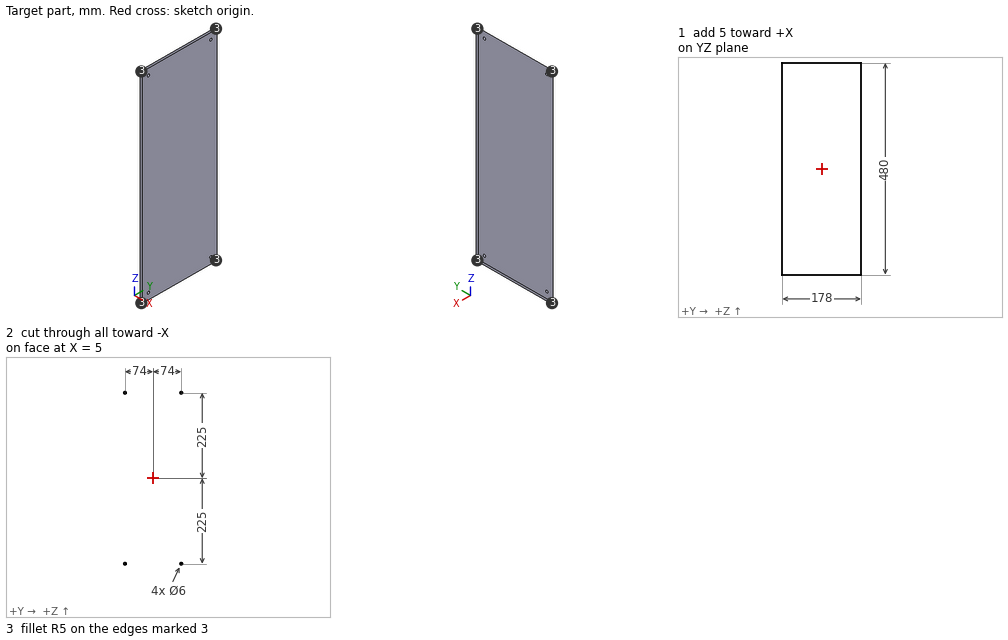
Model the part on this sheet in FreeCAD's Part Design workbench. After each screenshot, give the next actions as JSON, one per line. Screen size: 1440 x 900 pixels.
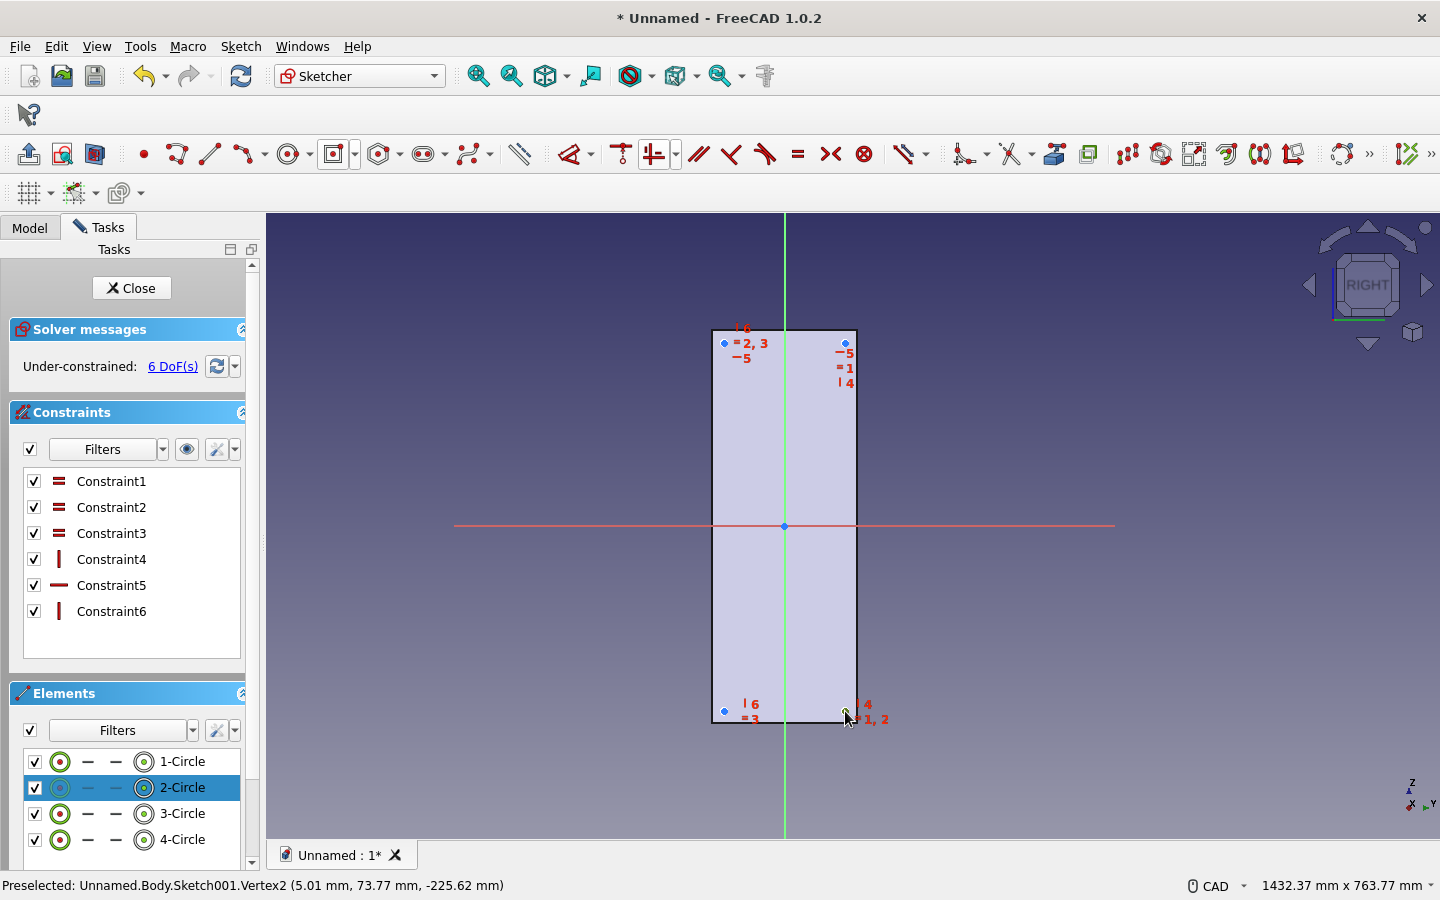
{"action": "left_click", "coordinate": [724, 711]}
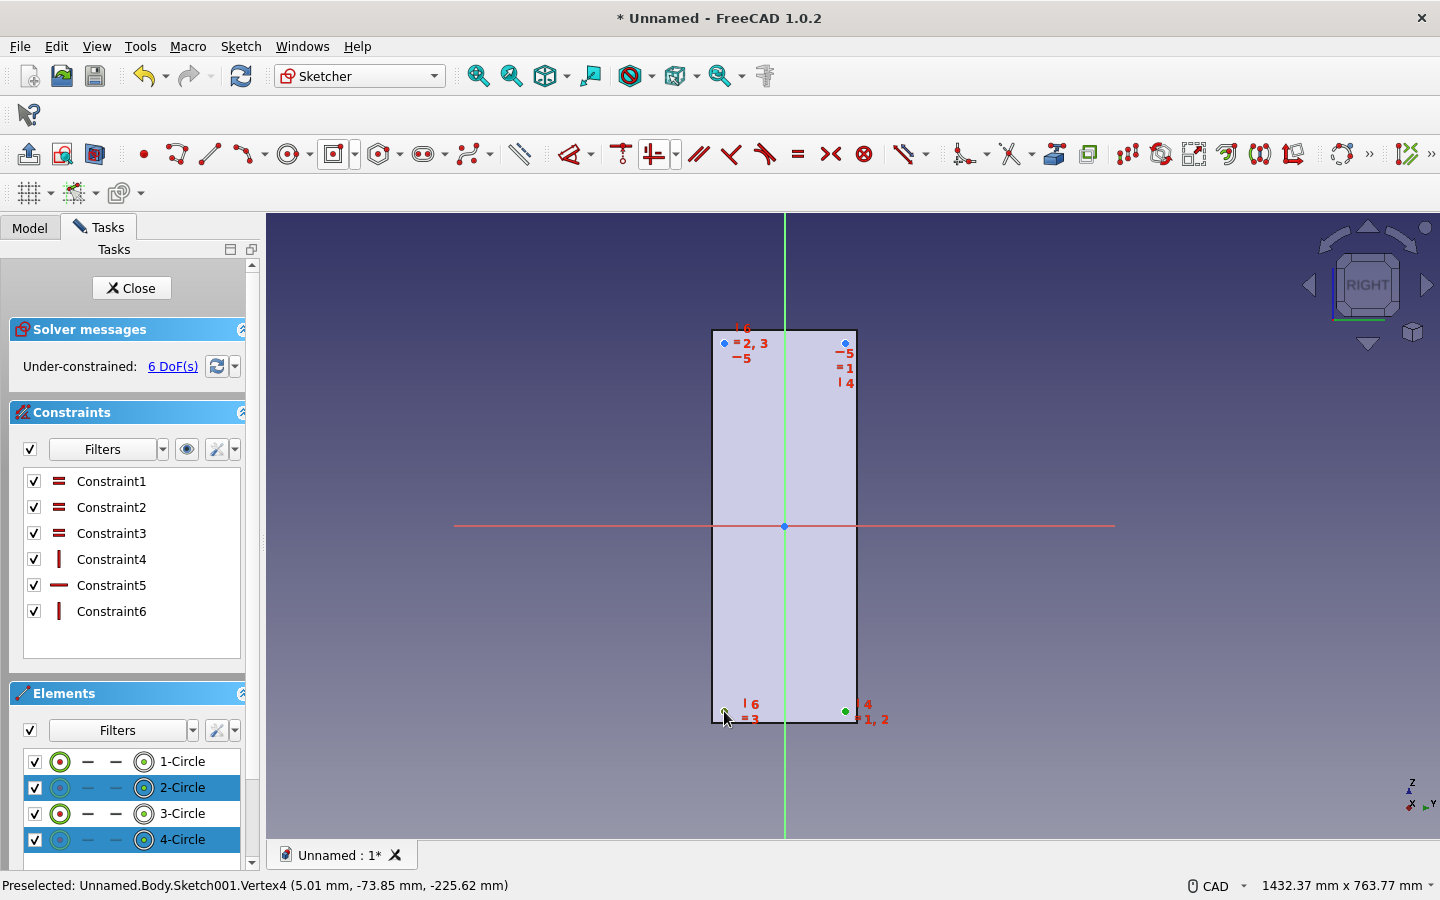
{"action": "key", "text": "h"}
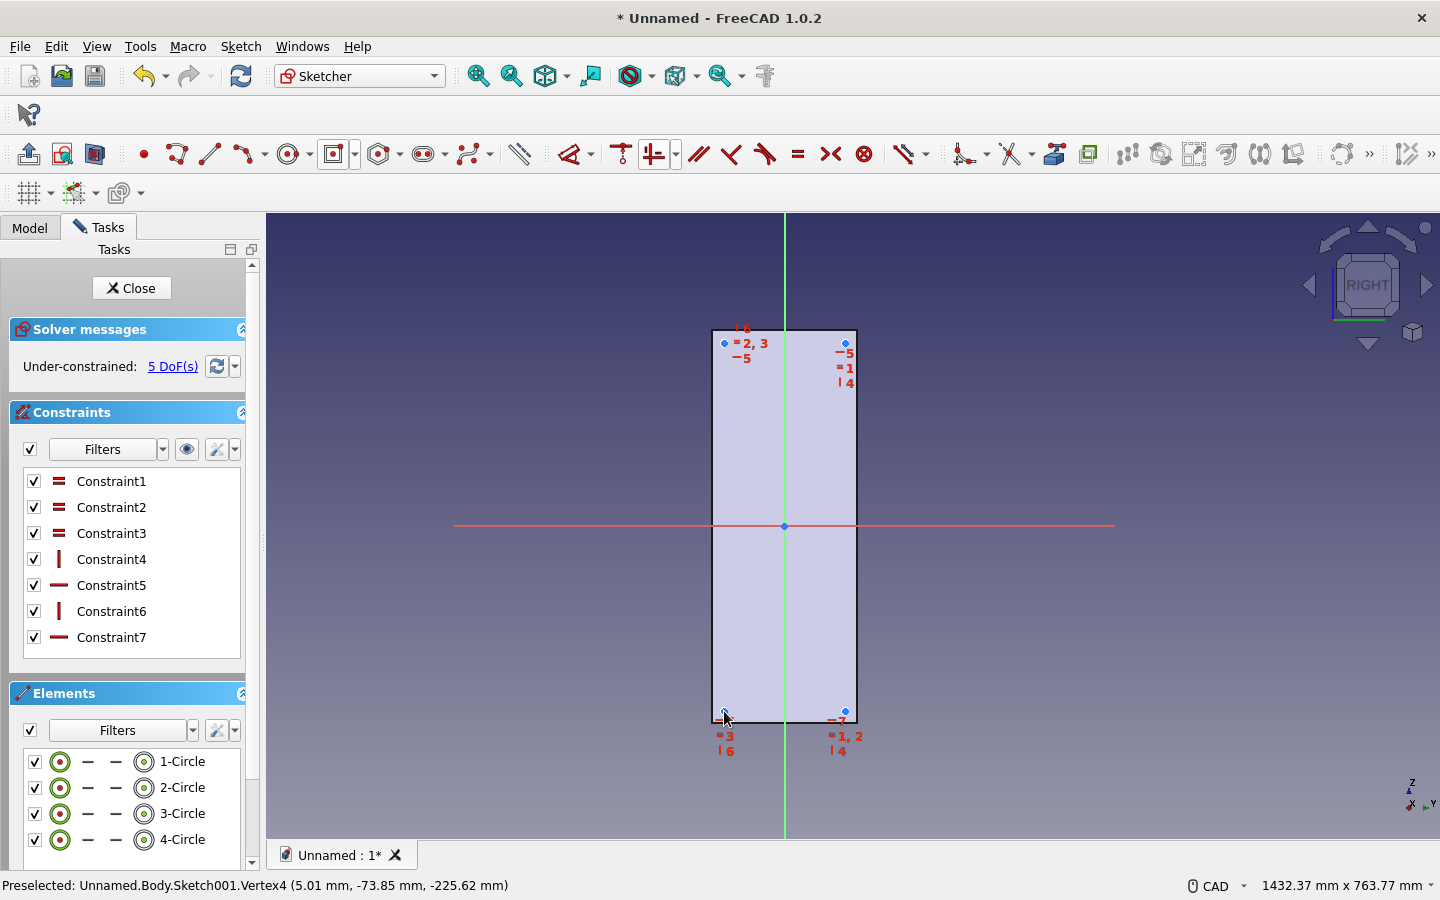
{"action": "scroll", "coordinate": [845, 340], "scroll_direction": "up", "scroll_amount": 11}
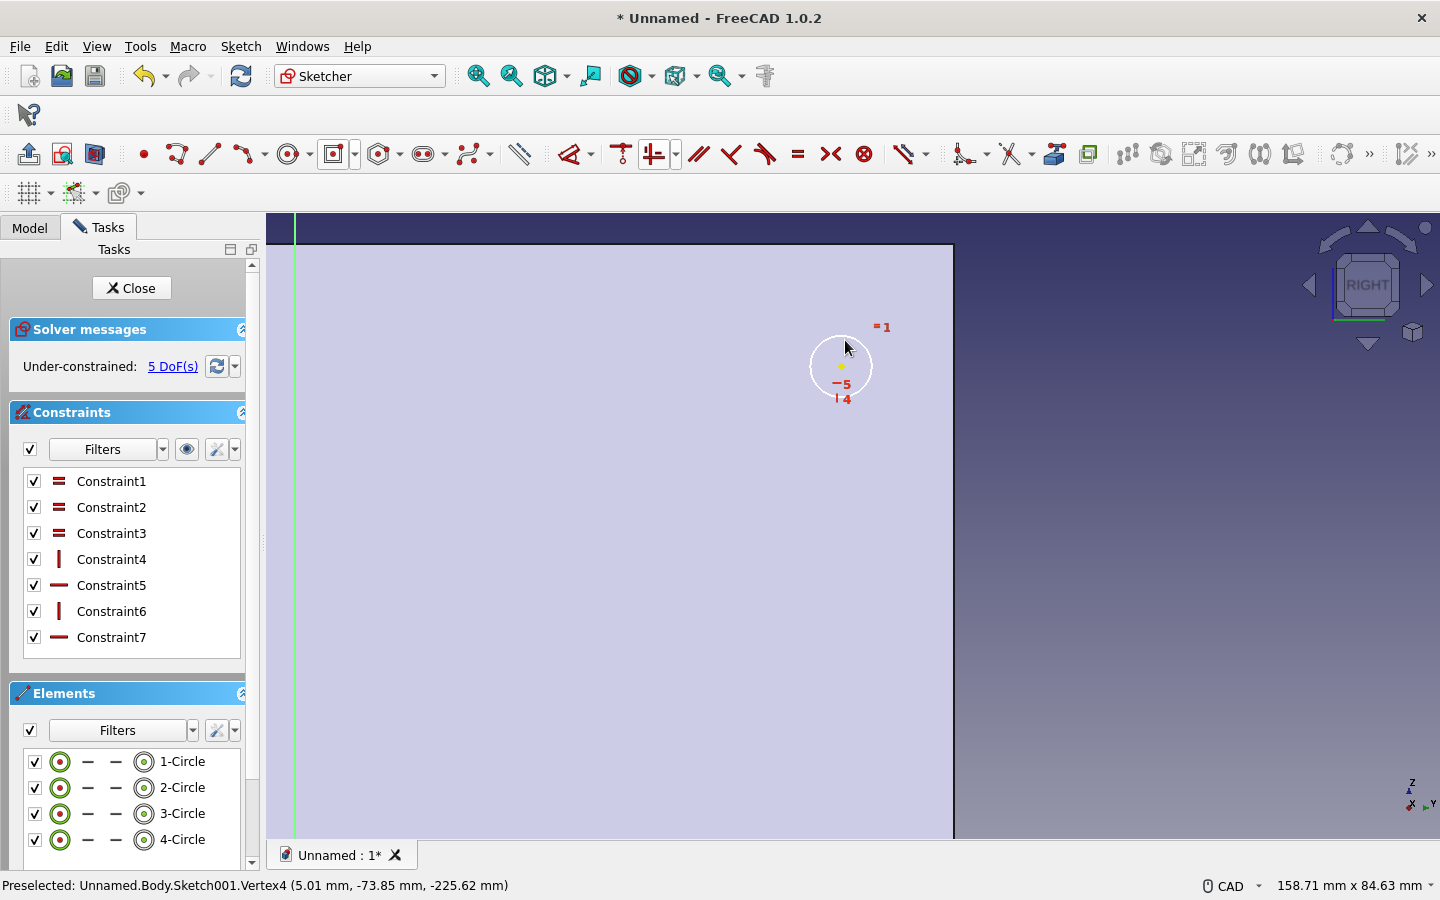
{"action": "left_click", "coordinate": [842, 336]}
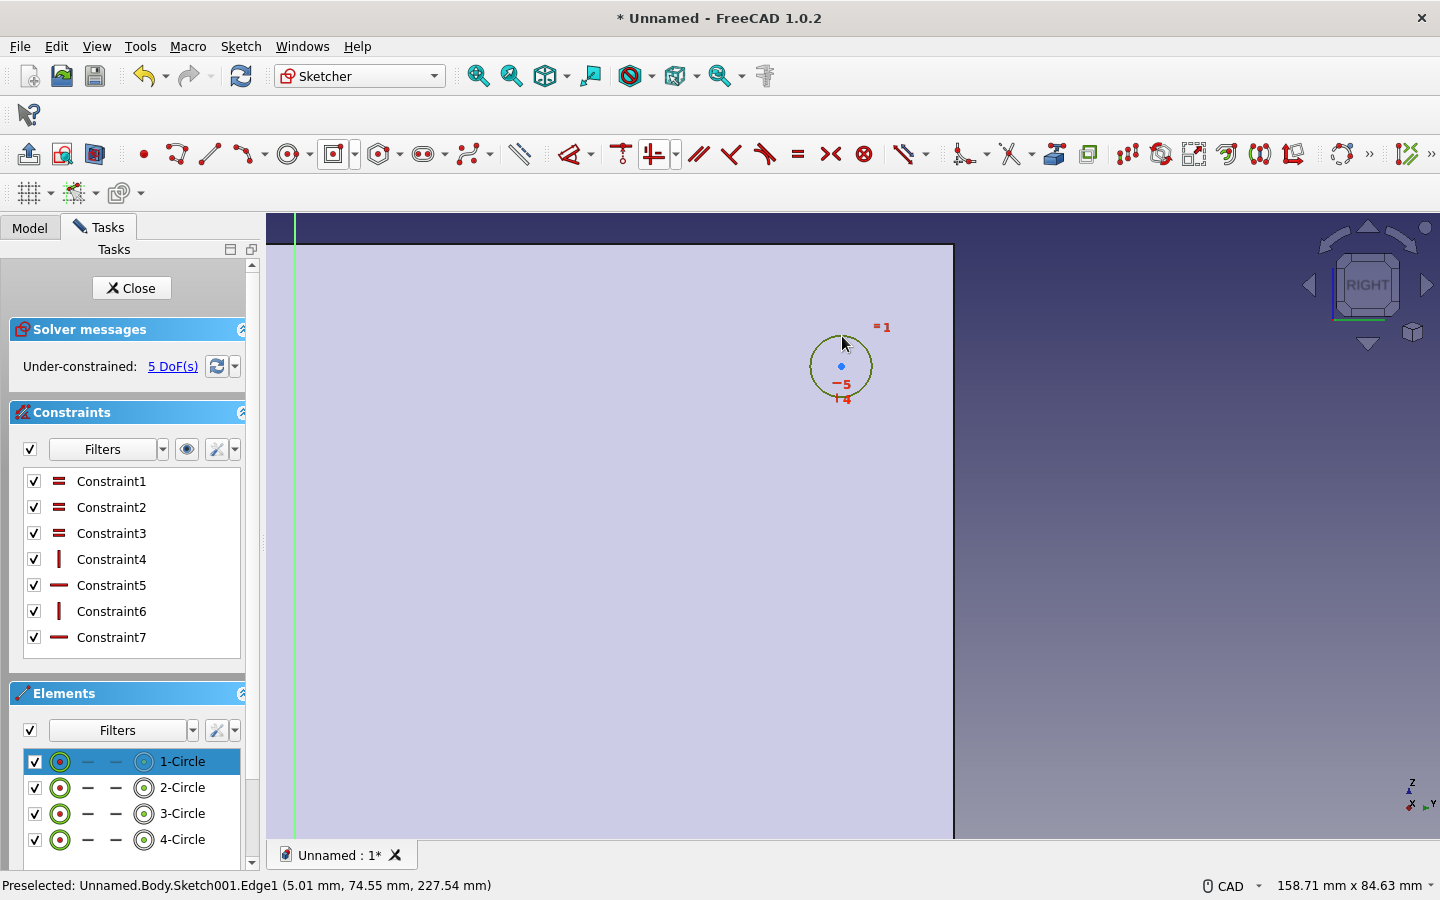
{"action": "left_click", "coordinate": [590, 154]}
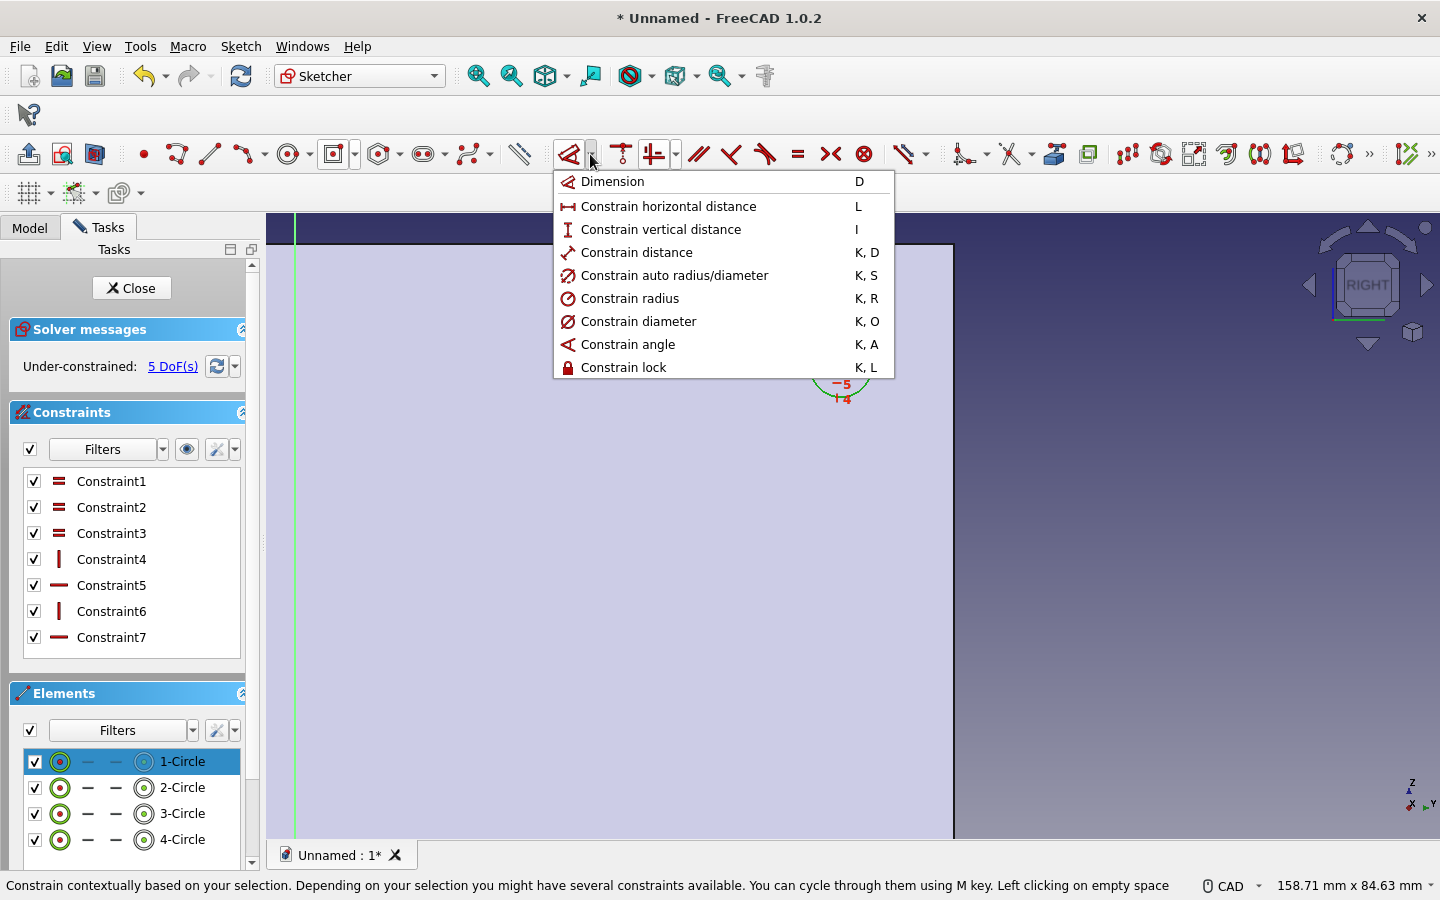
{"action": "left_click", "coordinate": [724, 322]}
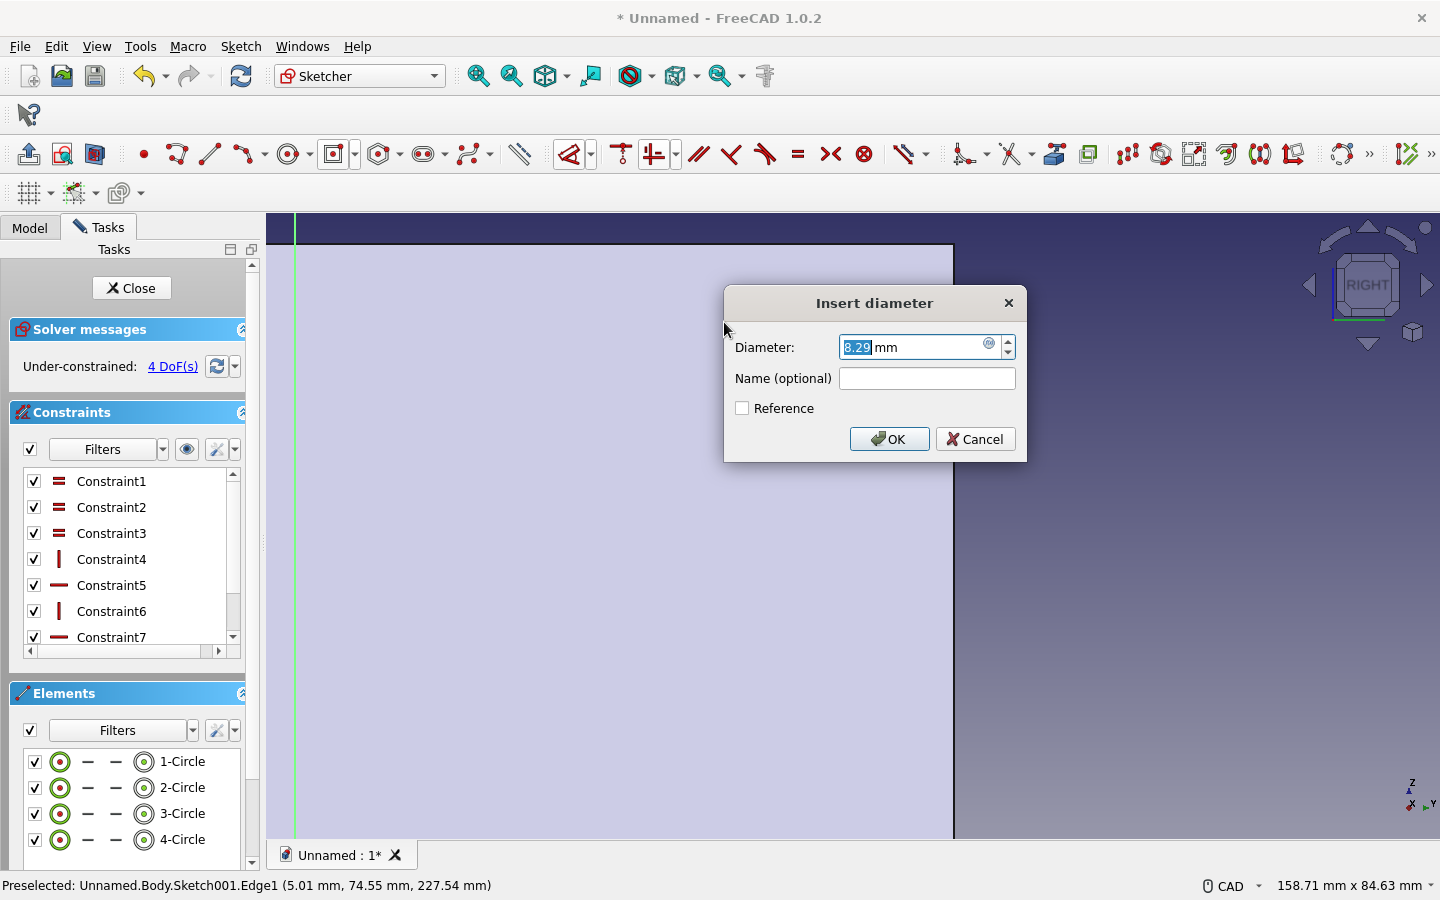
{"action": "type", "text": "6"}
{"action": "key", "text": "Return"}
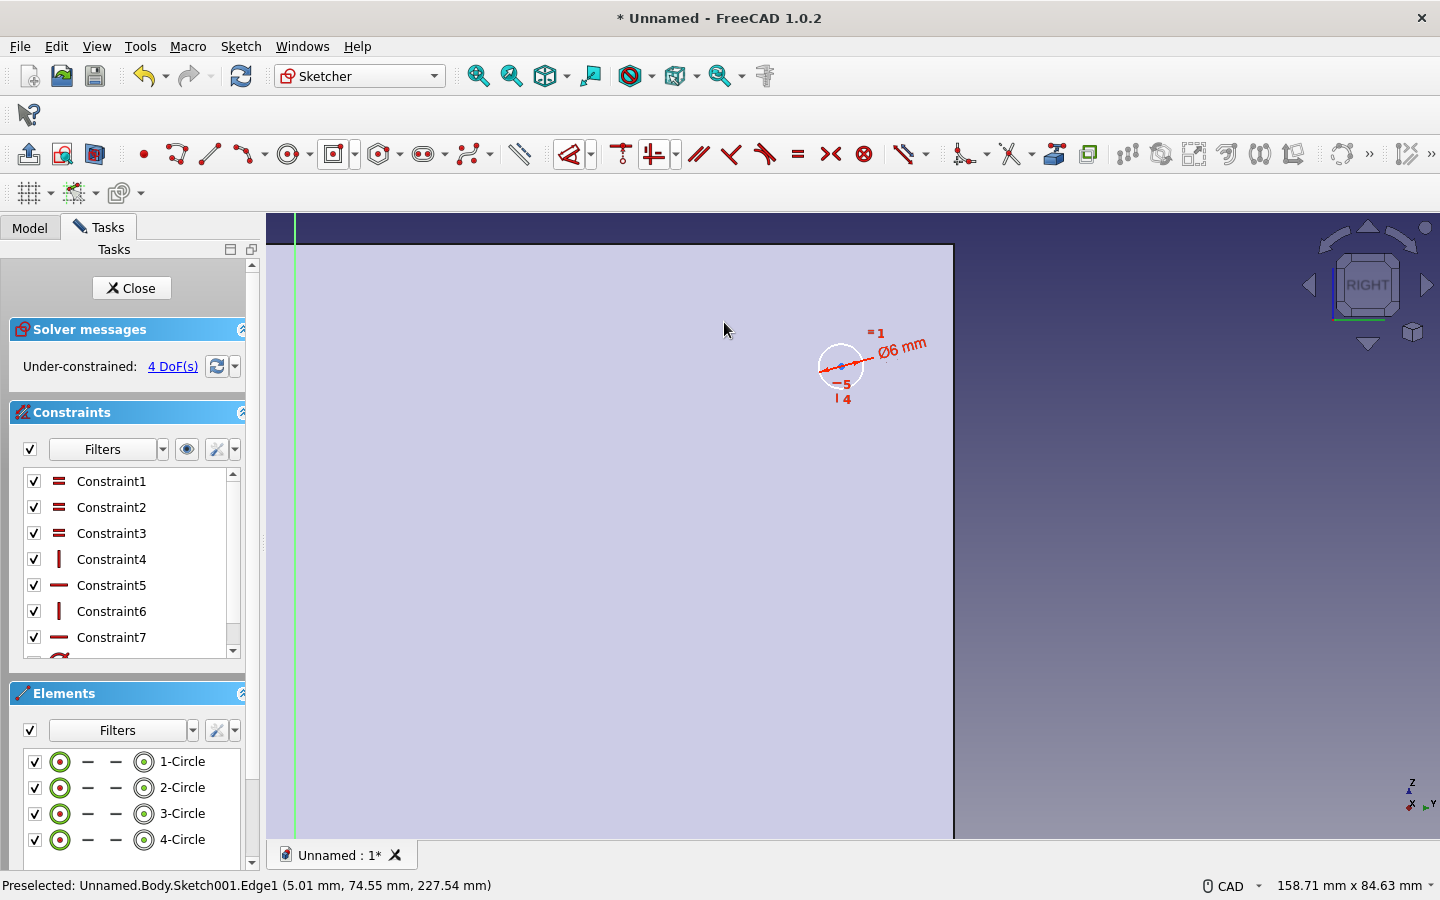
{"action": "scroll", "coordinate": [845, 340], "scroll_direction": "down", "scroll_amount": 11}